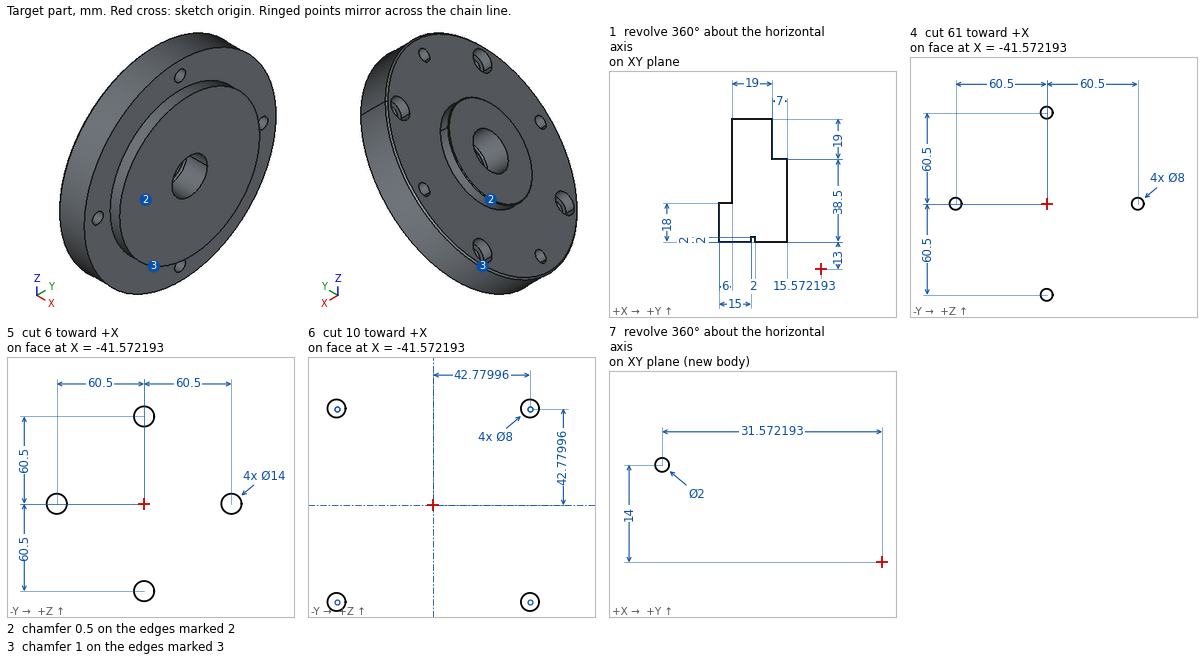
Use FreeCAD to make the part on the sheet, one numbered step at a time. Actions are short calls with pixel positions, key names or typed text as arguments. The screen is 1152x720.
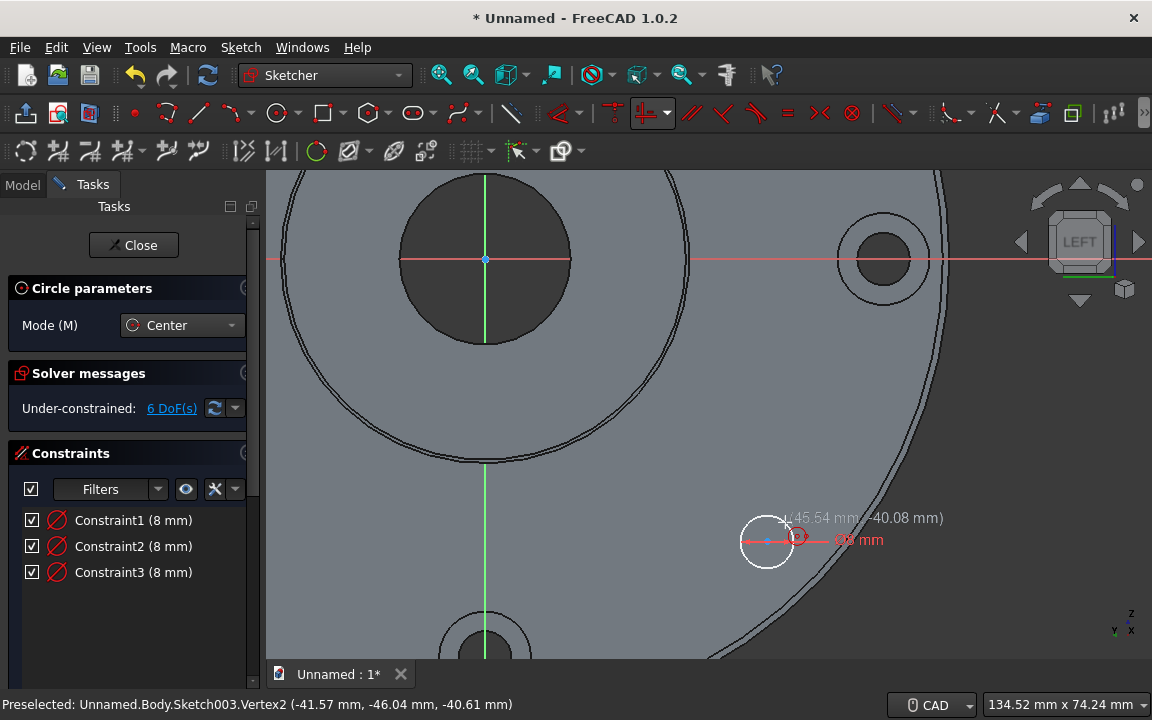
scroll(767, 541, down, 4)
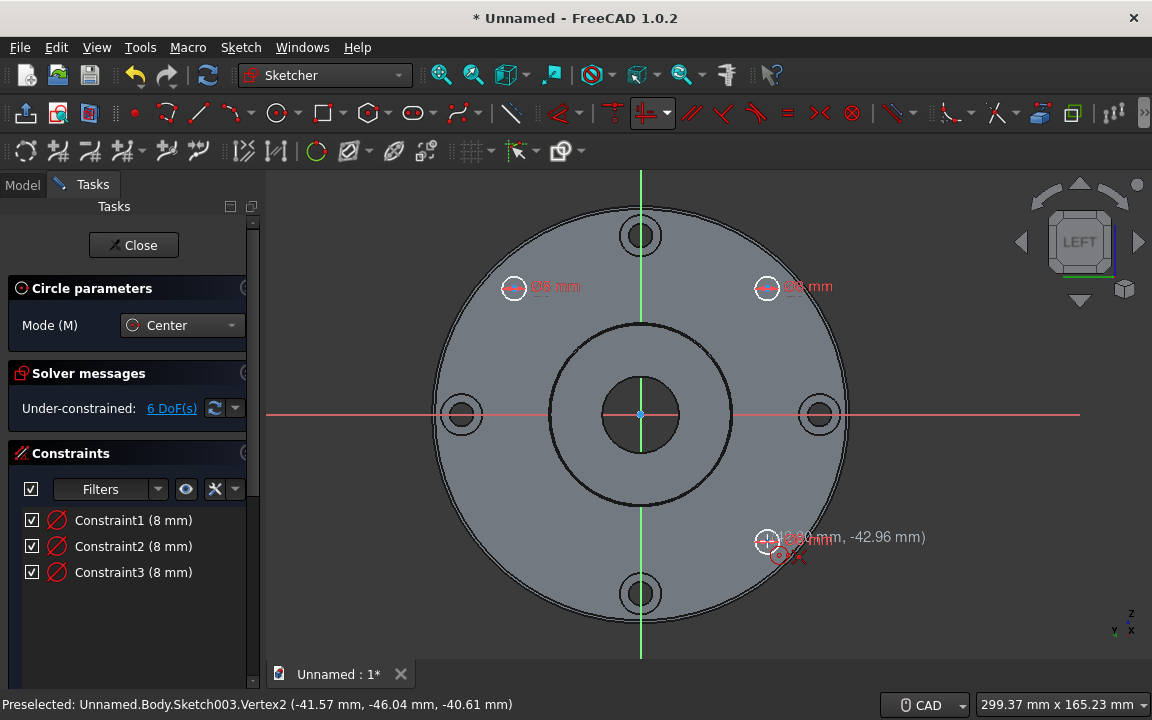
scroll(514, 541, up, 4)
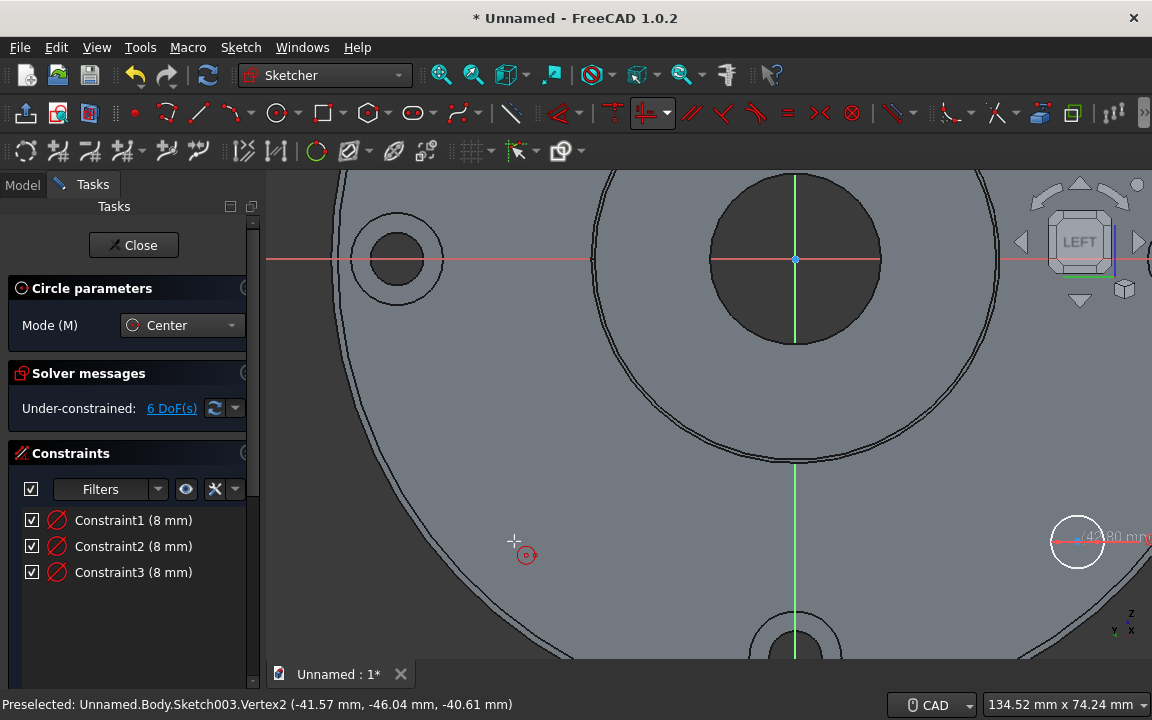
click(514, 541)
move(532, 522)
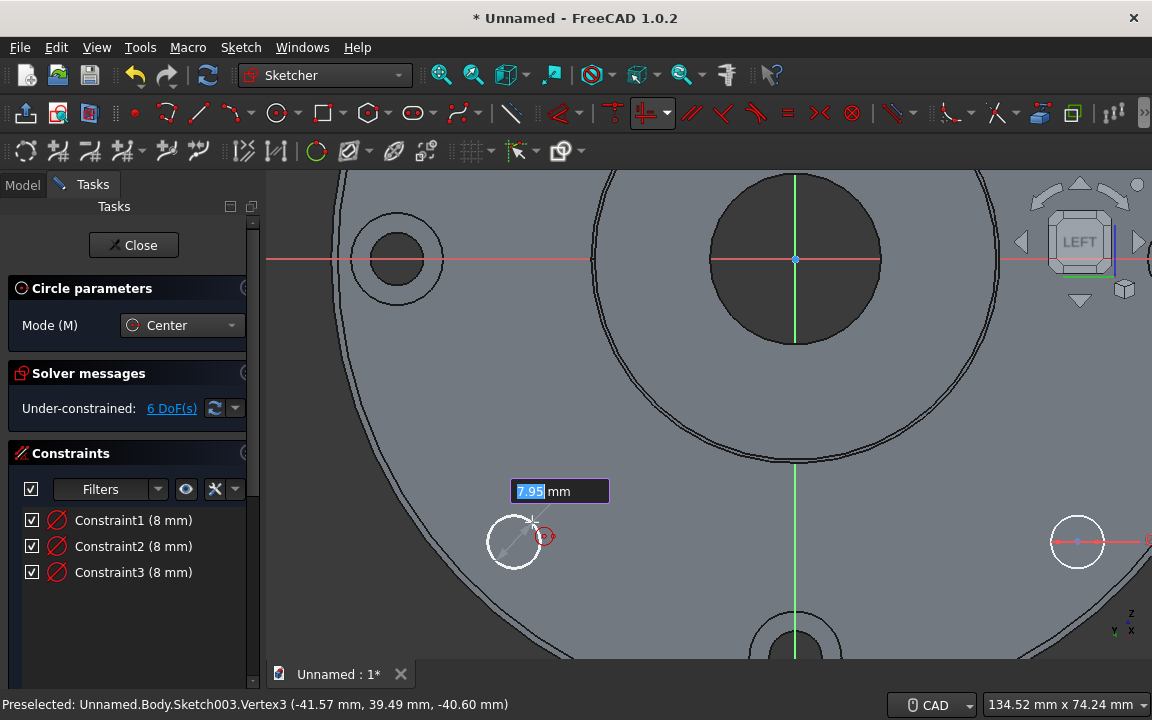
text(8)
key(Return)
key(Escape)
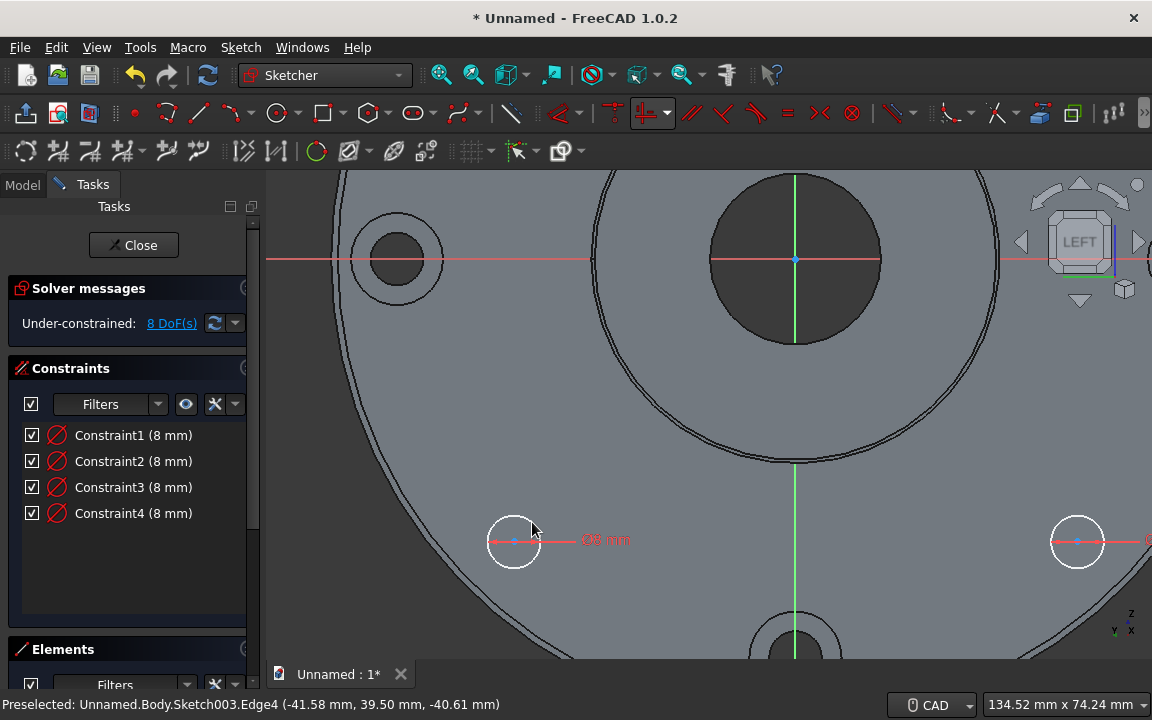
scroll(514, 541, down, 4)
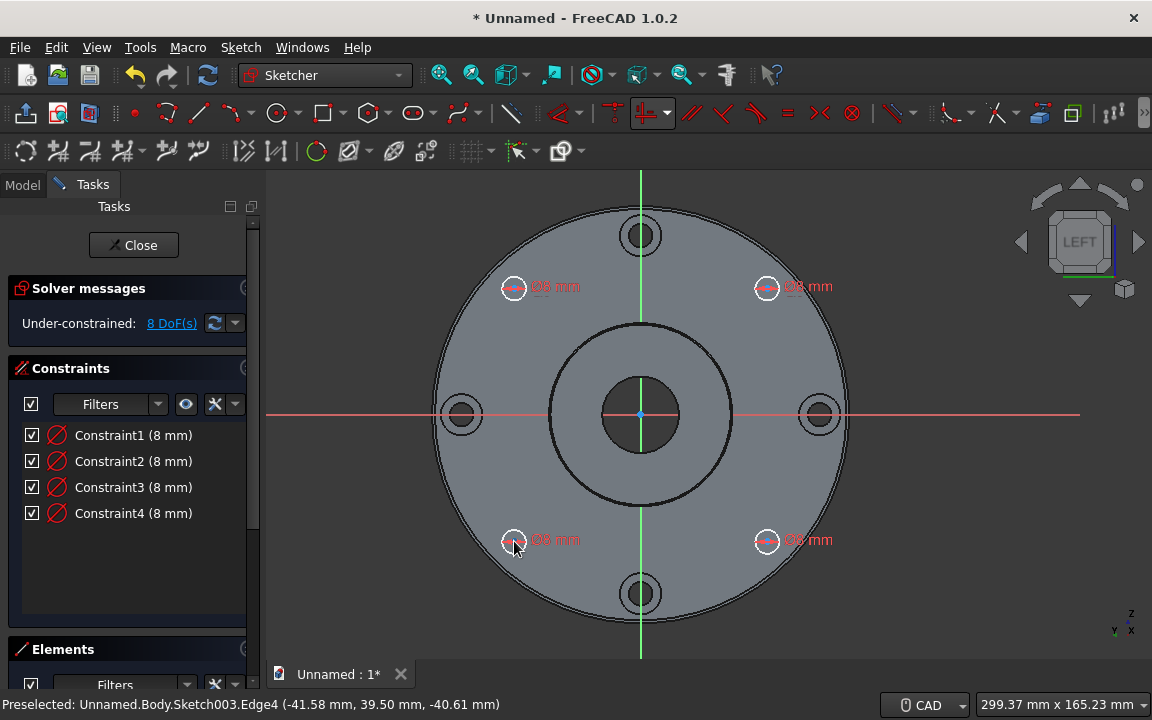
click(767, 289)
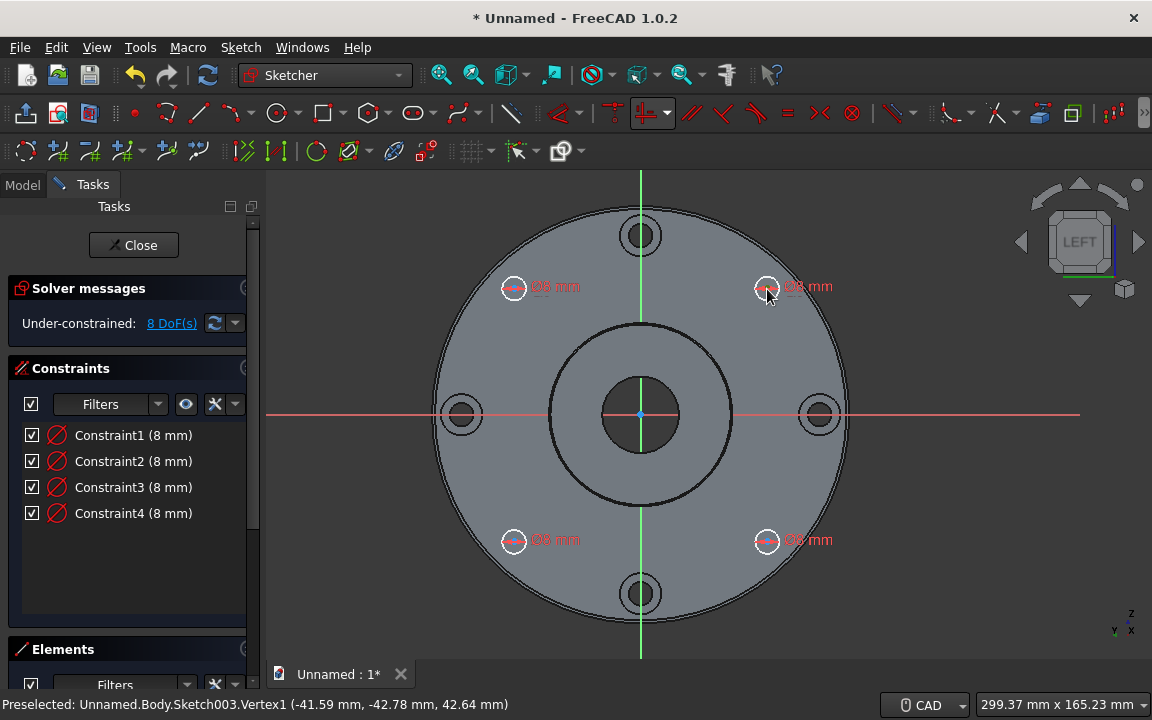
click(514, 289)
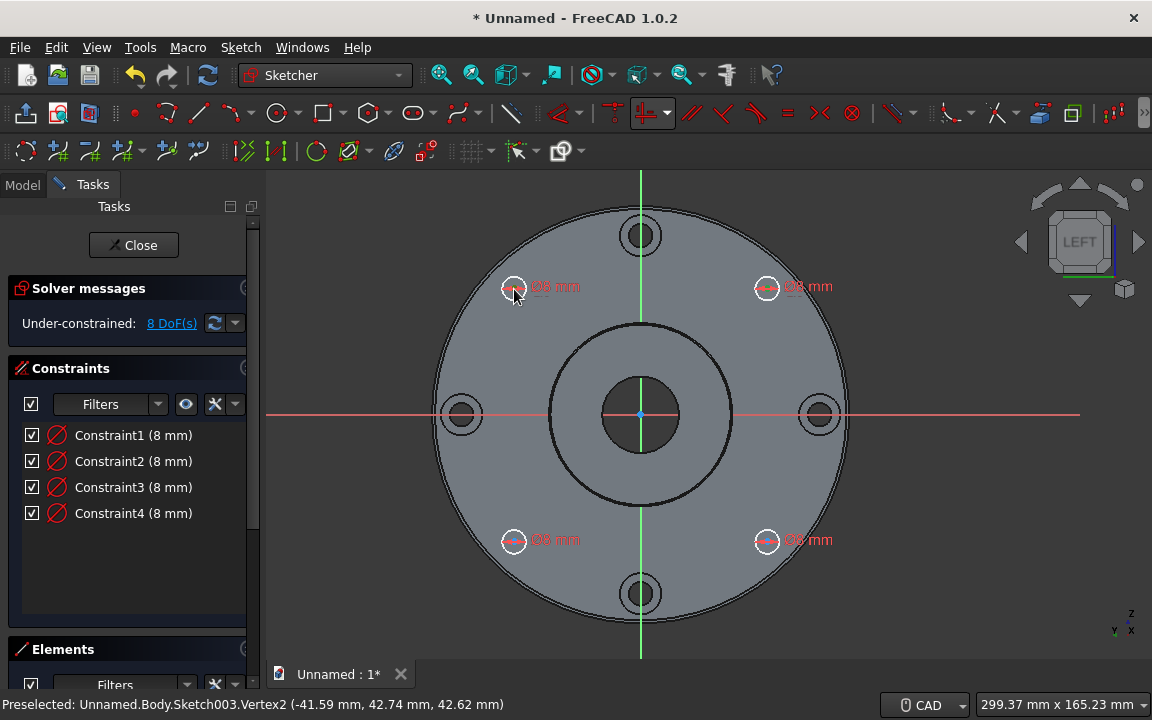
click(641, 600)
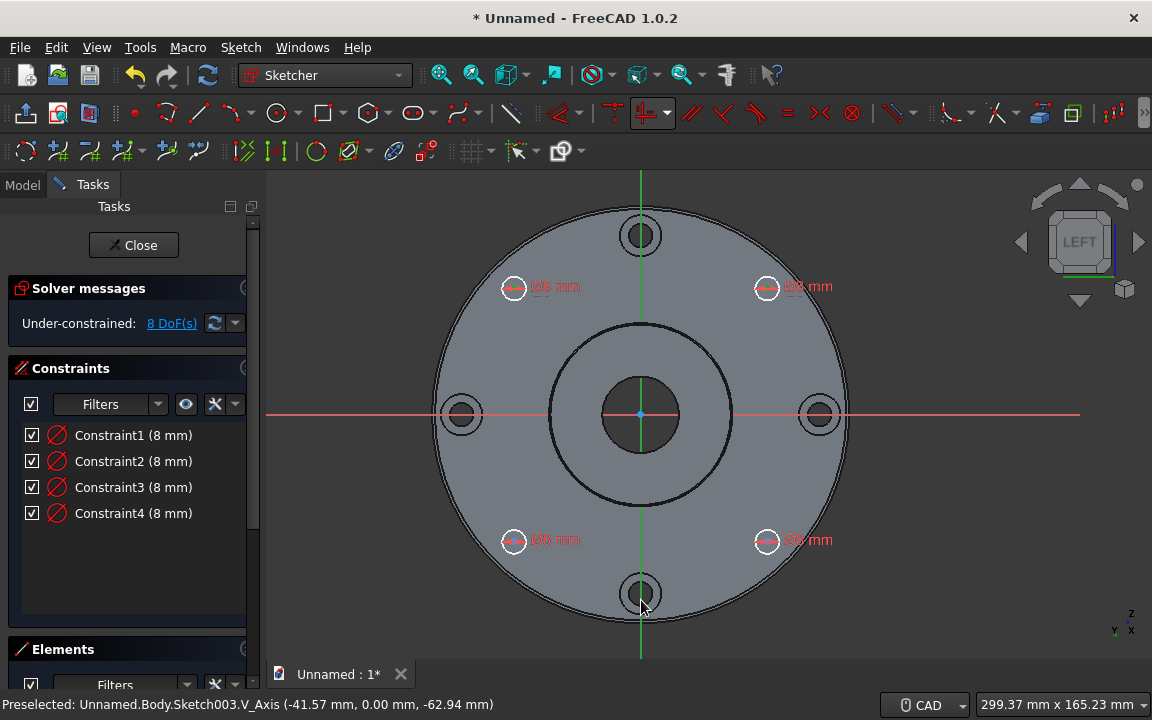
click(820, 114)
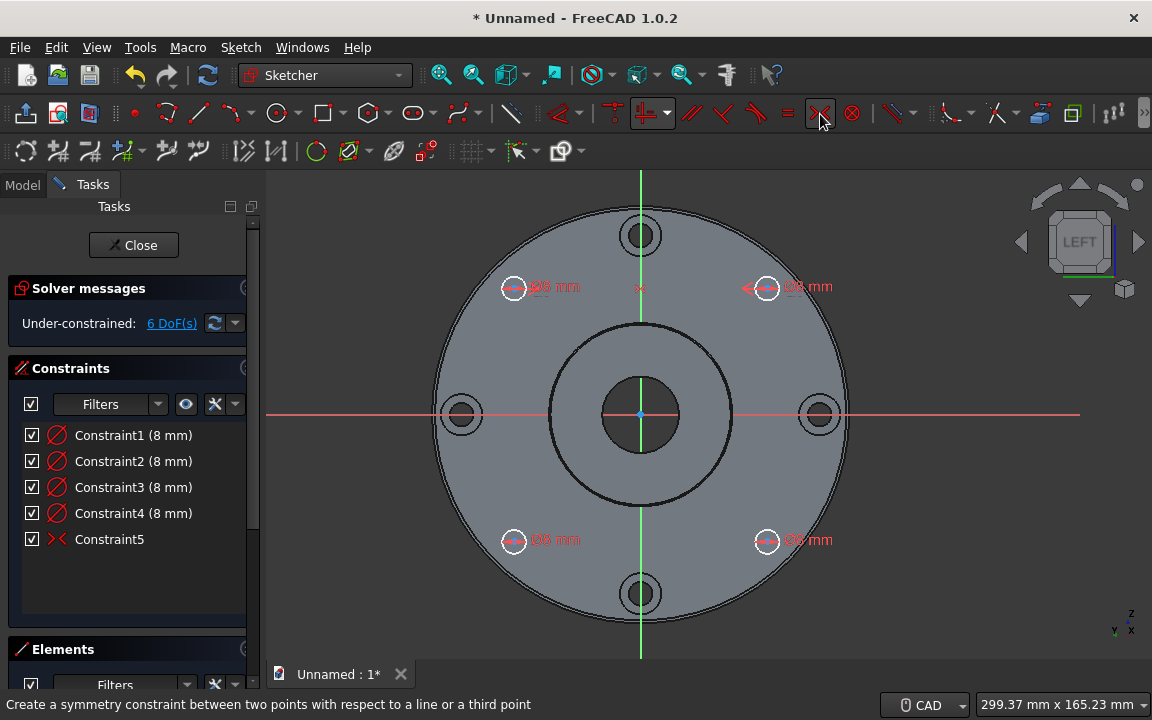
click(767, 289)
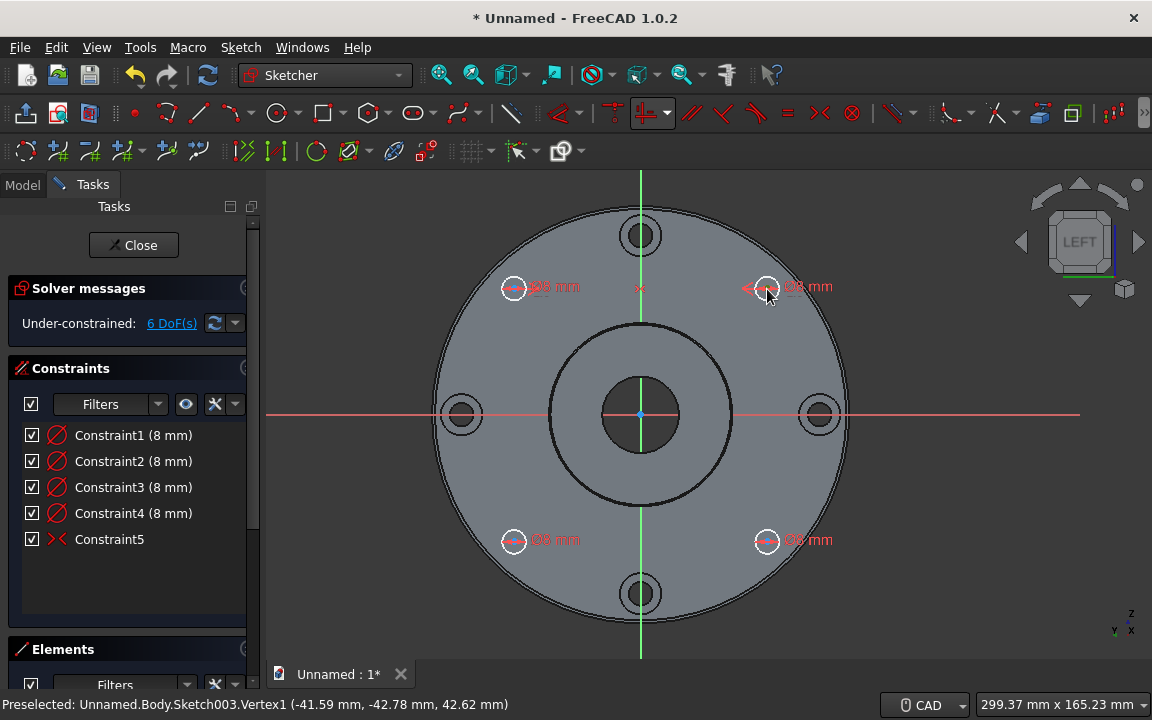
click(767, 542)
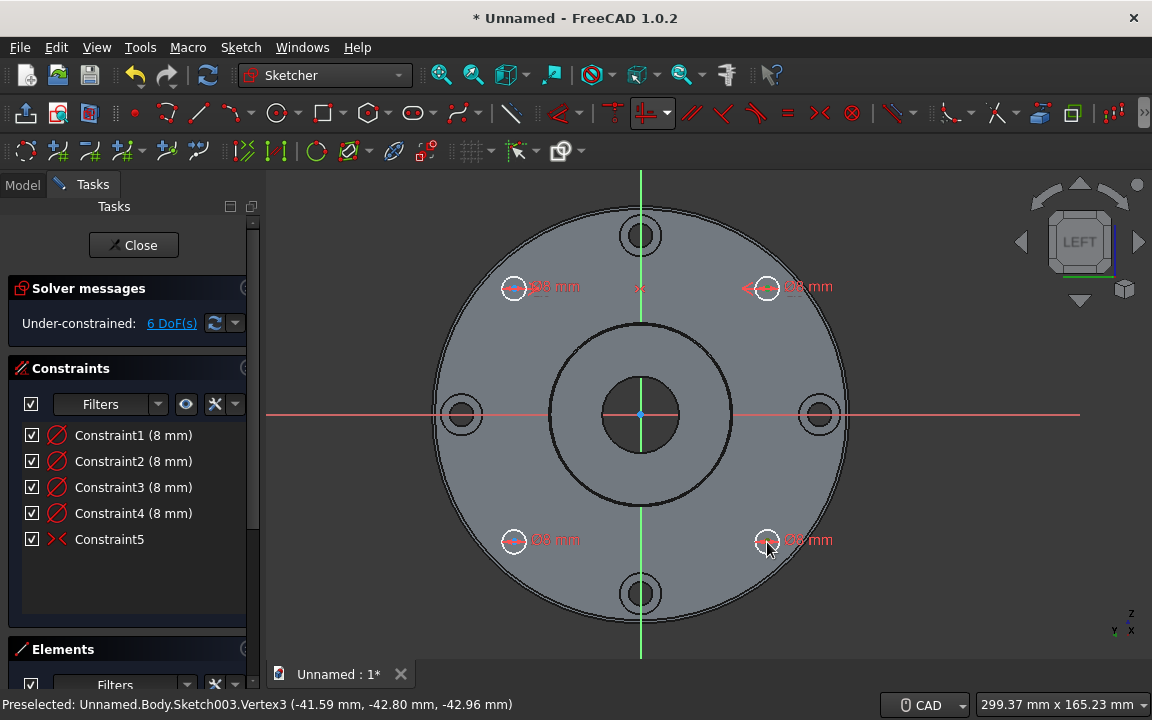
click(344, 415)